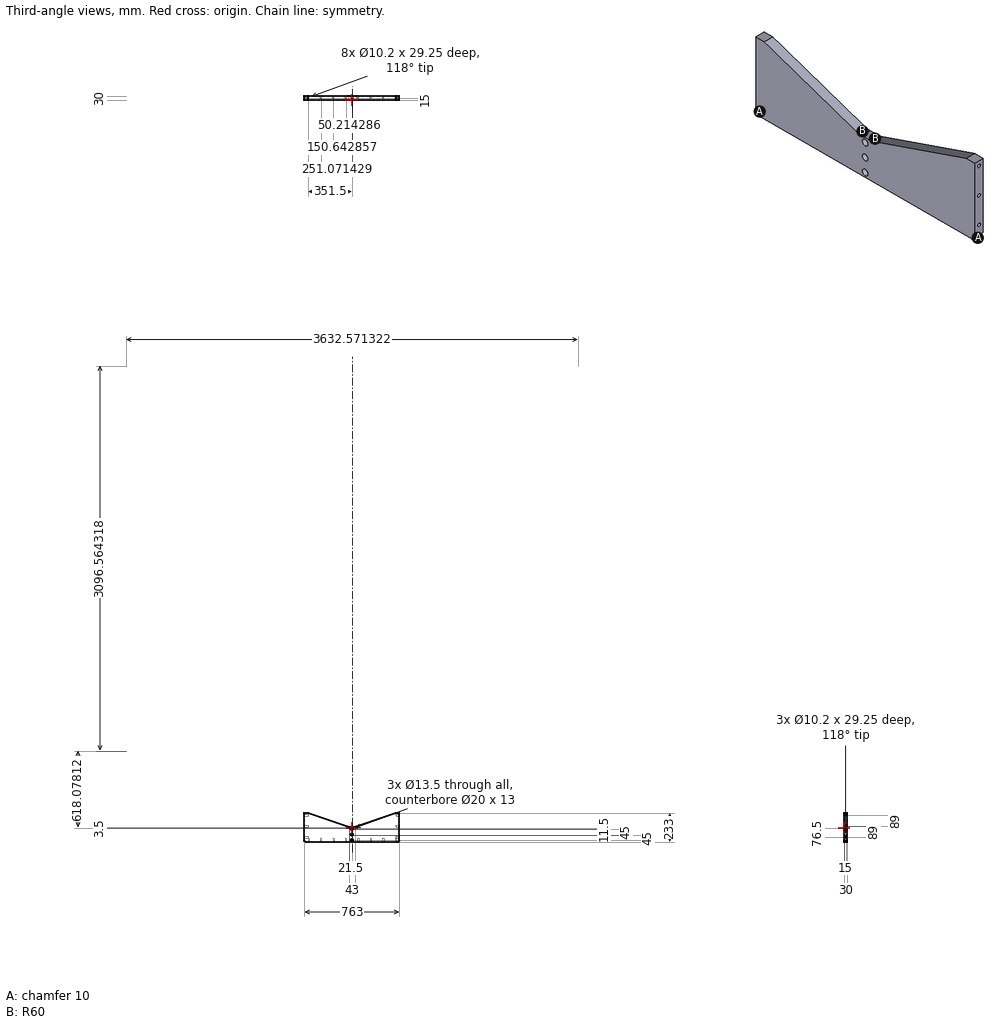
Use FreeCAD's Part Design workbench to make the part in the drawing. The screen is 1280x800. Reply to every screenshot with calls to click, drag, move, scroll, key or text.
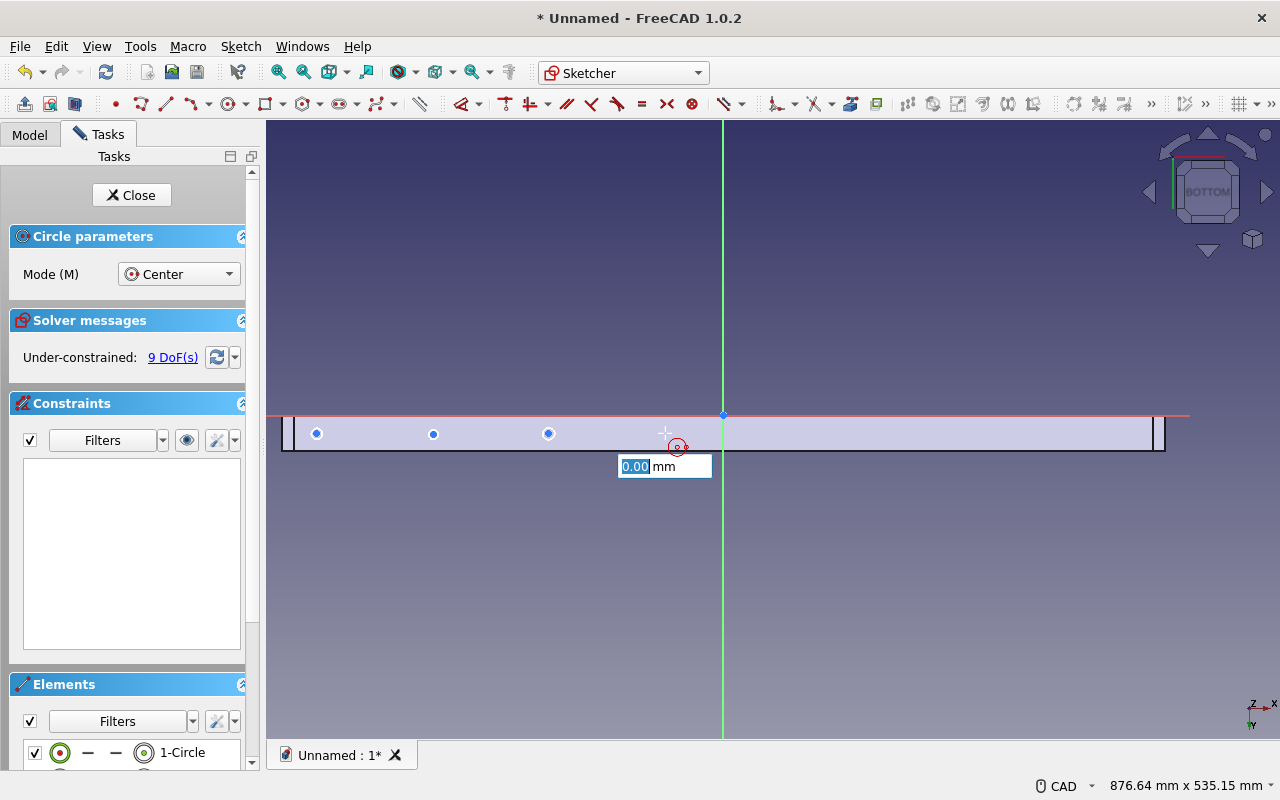
scroll(669, 437, up, 5)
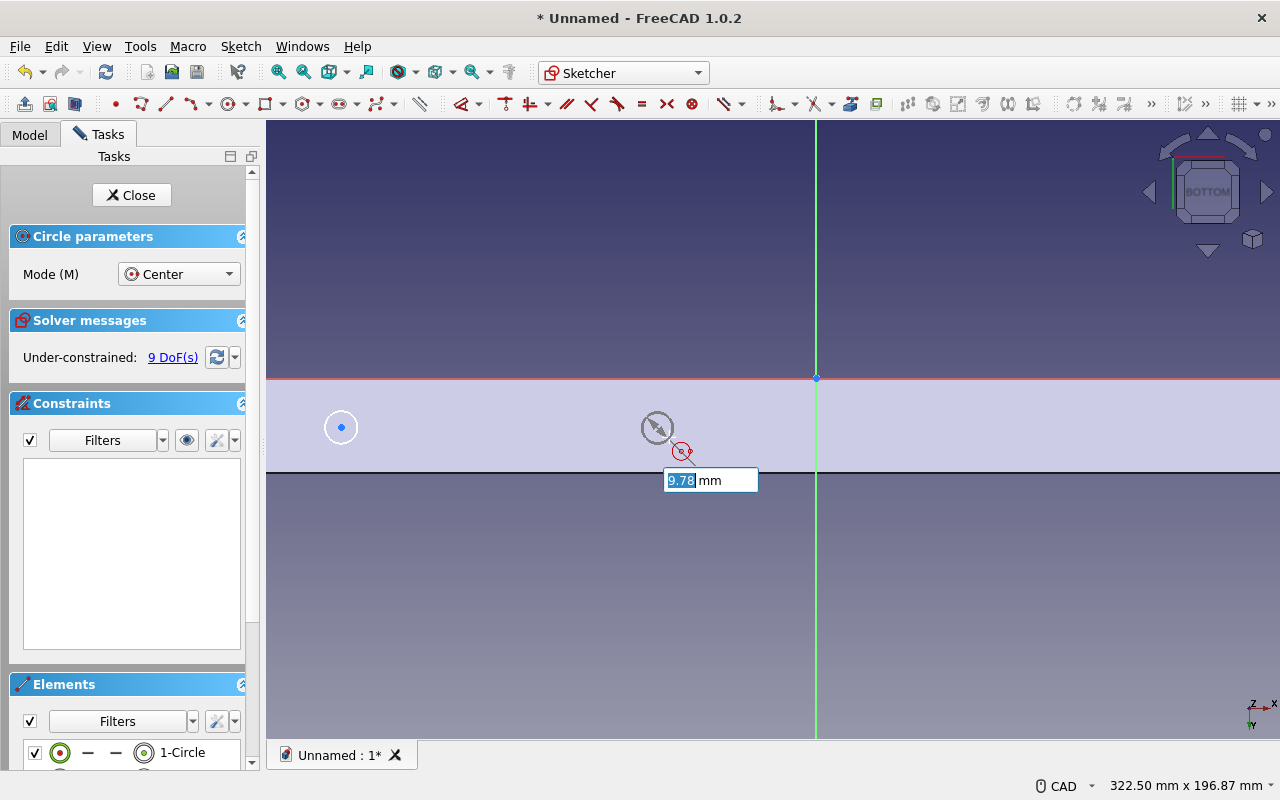
click(670, 437)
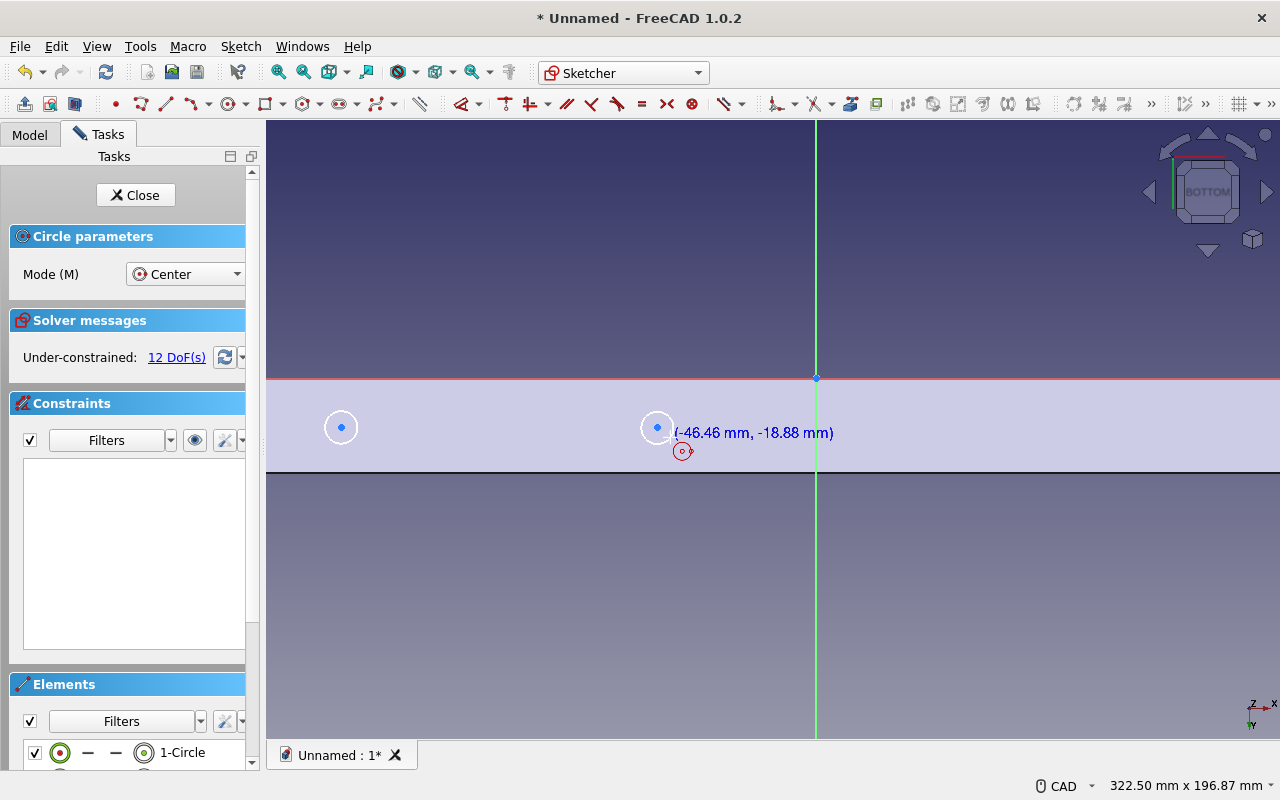
scroll(974, 426, up, 2)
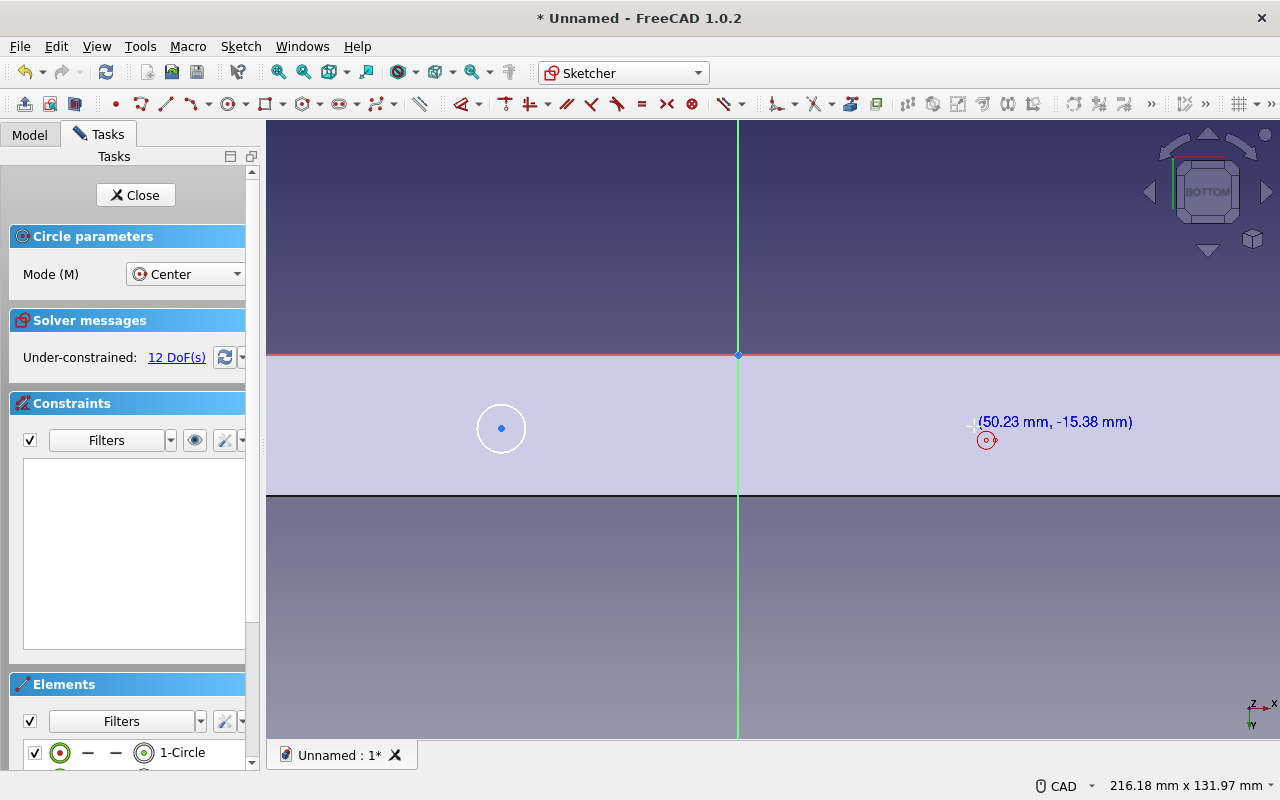
scroll(698, 435, down, 9)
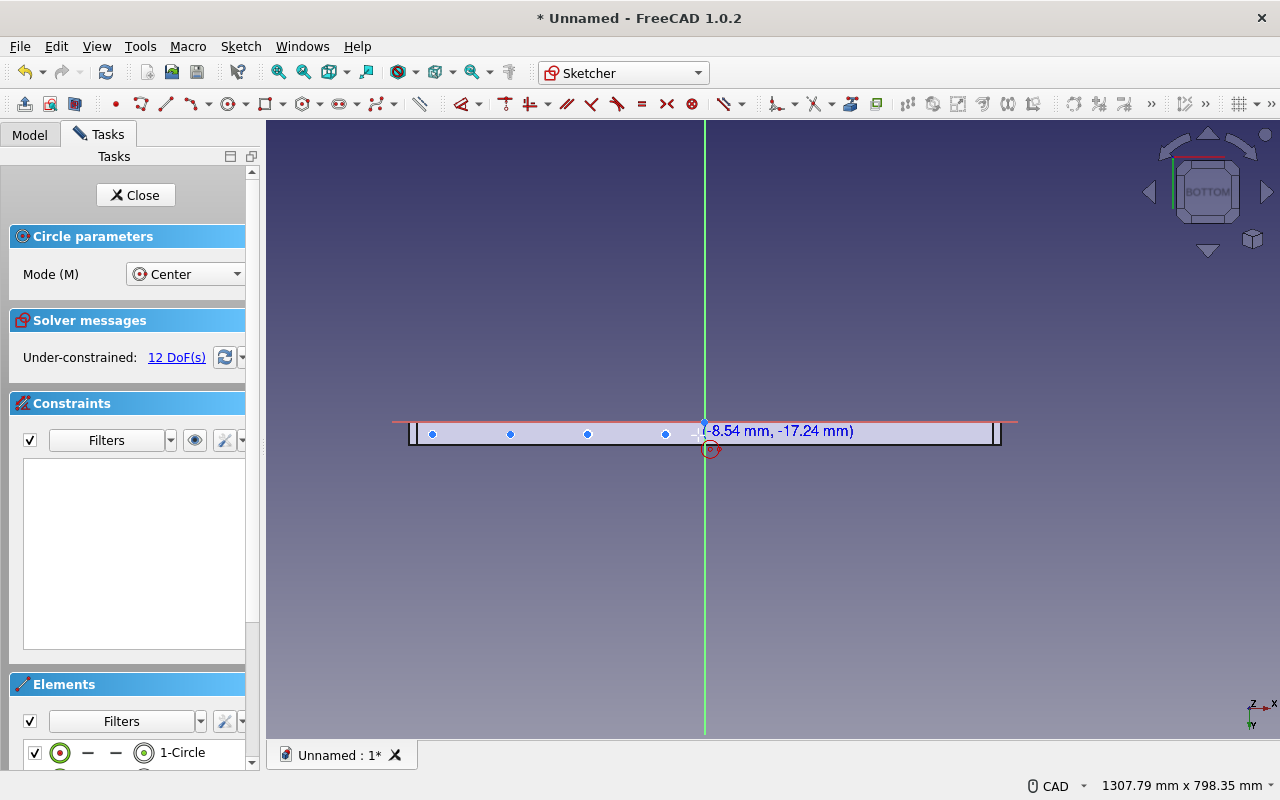
scroll(744, 434, up, 2)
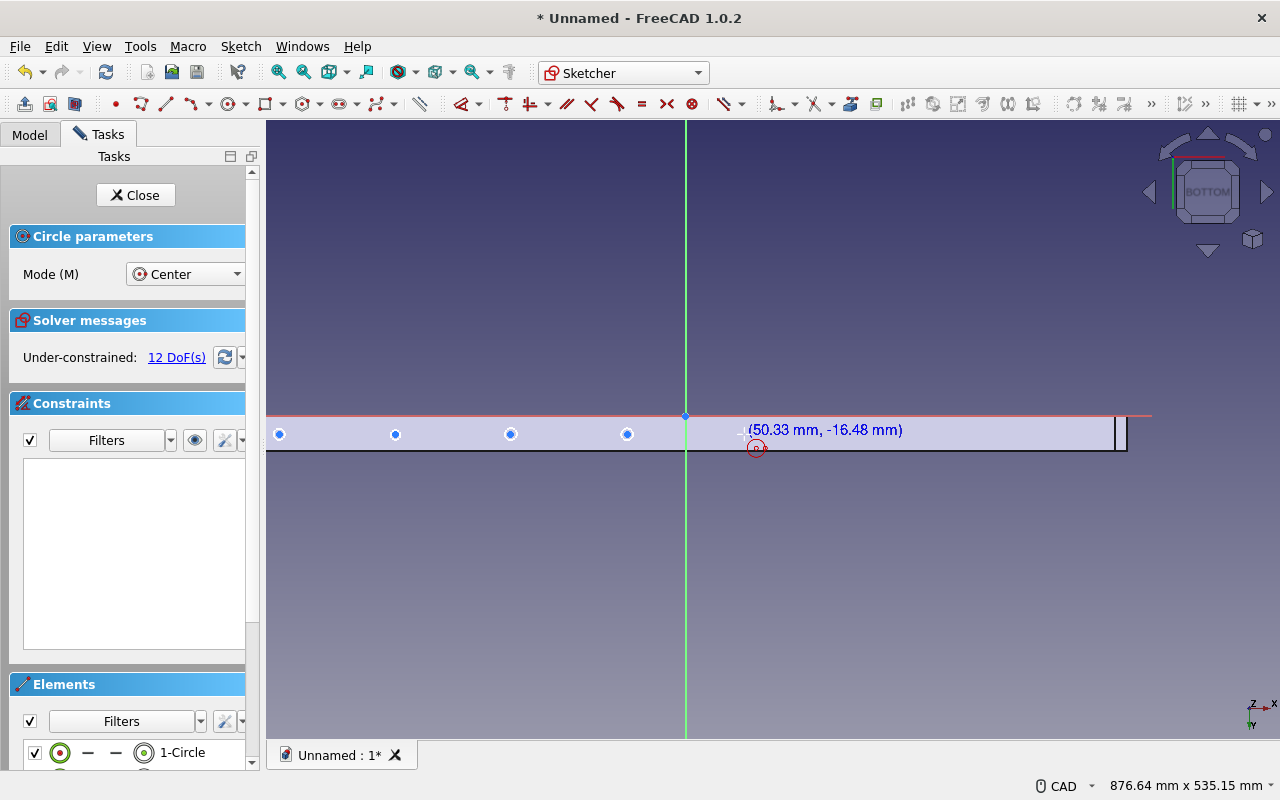
click(744, 434)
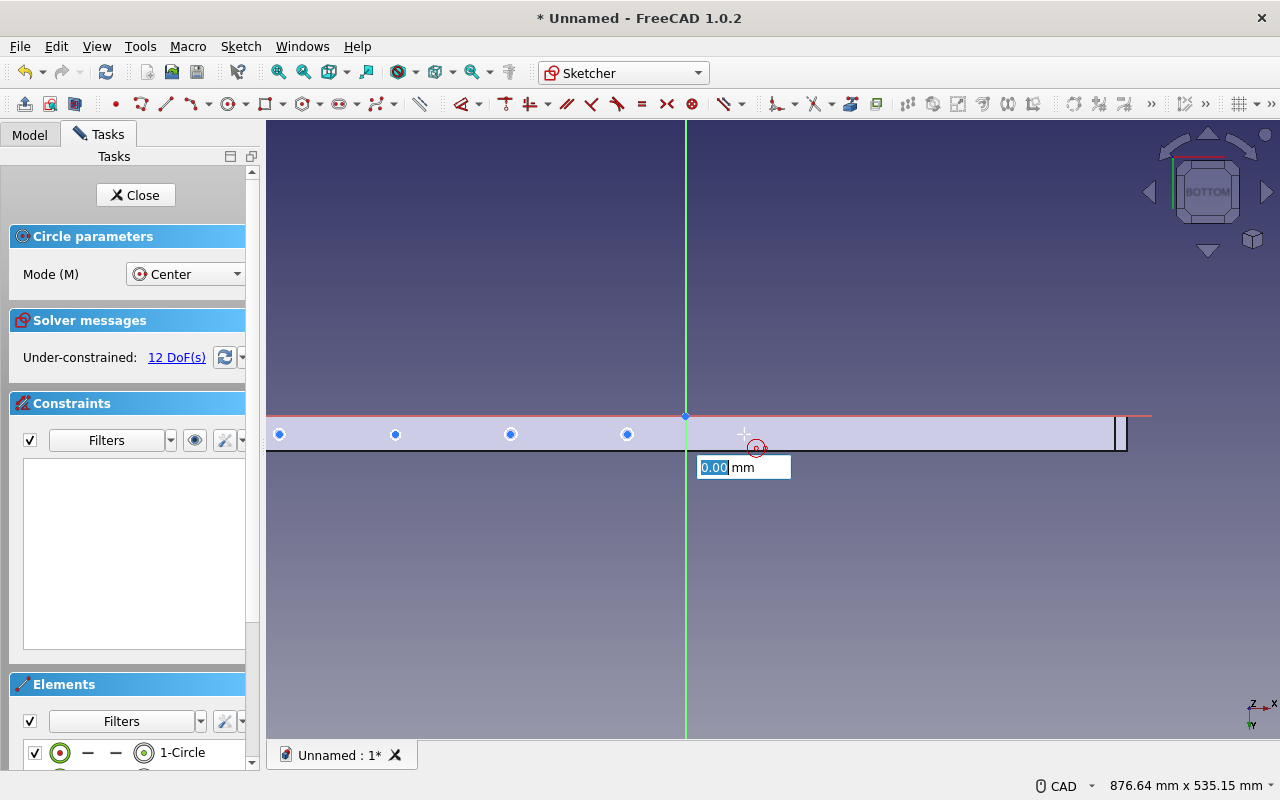
scroll(748, 438, up, 5)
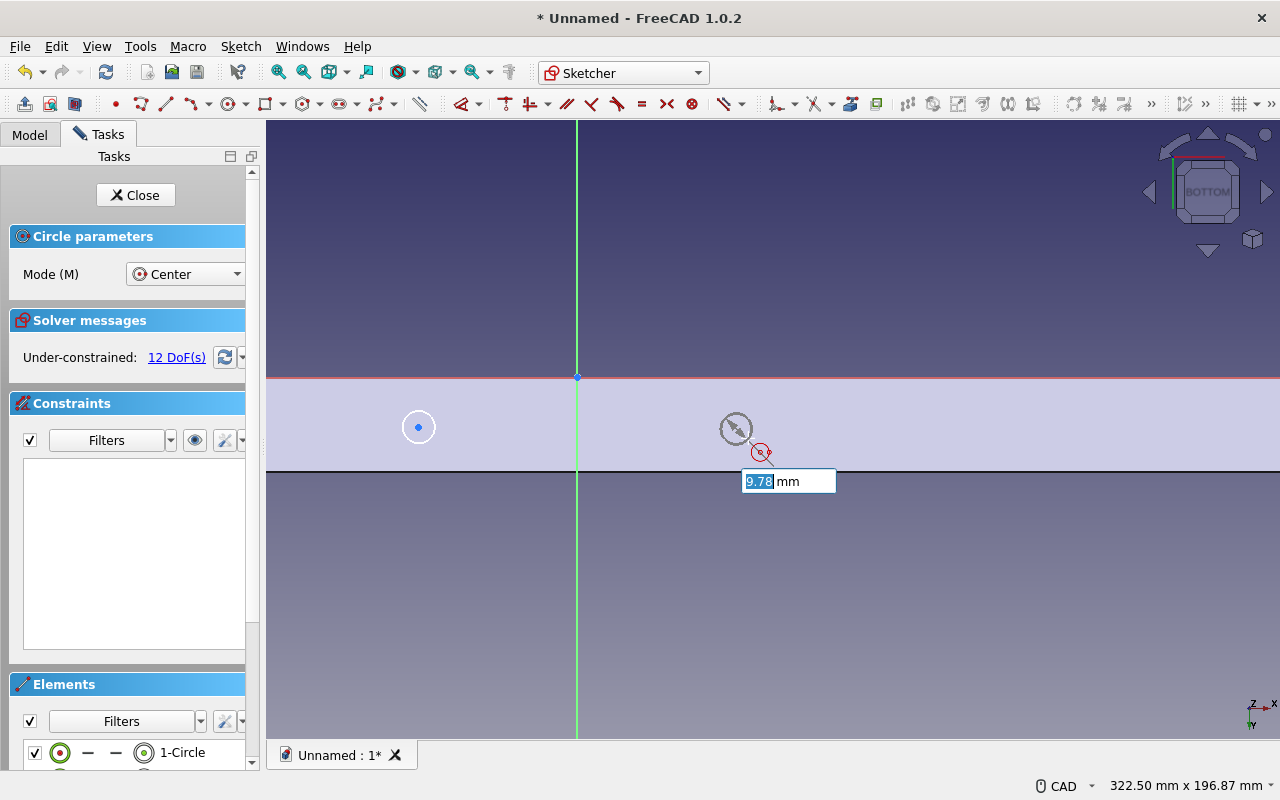
click(747, 436)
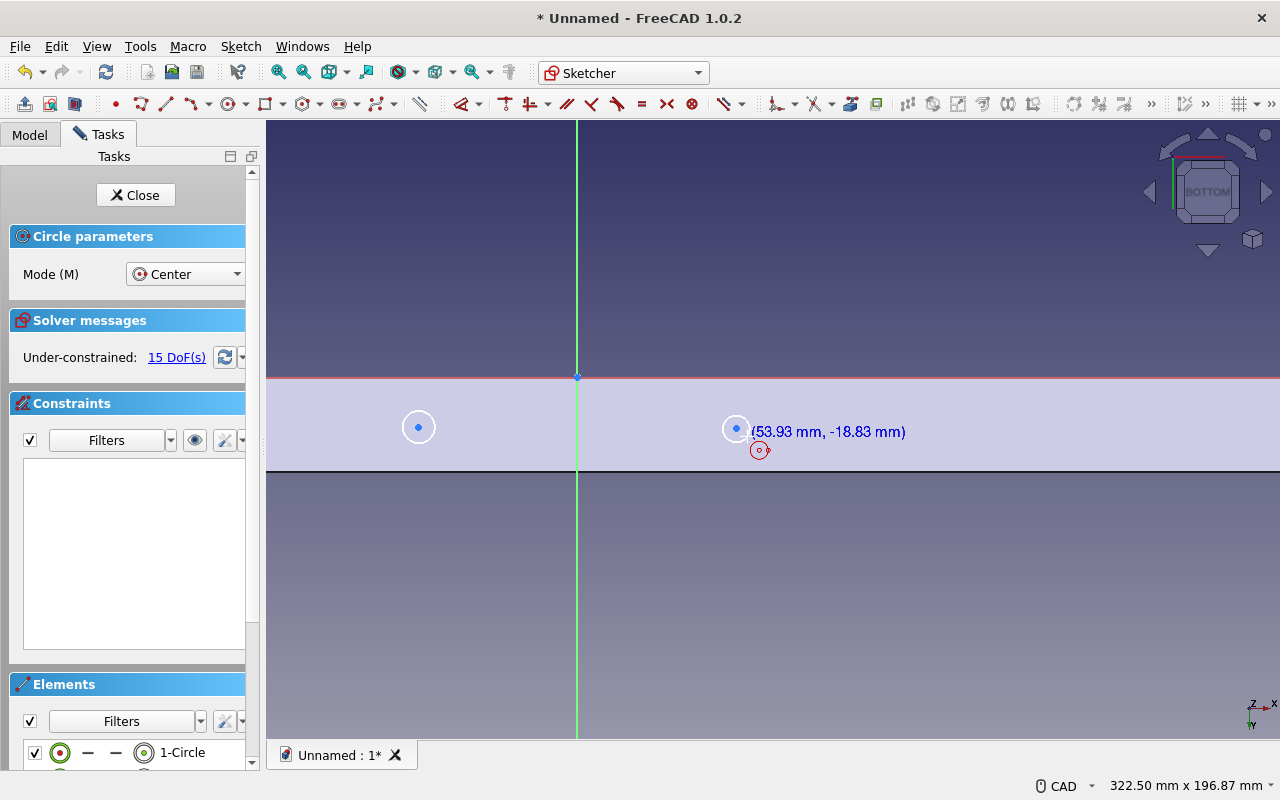
scroll(1051, 425, up, 2)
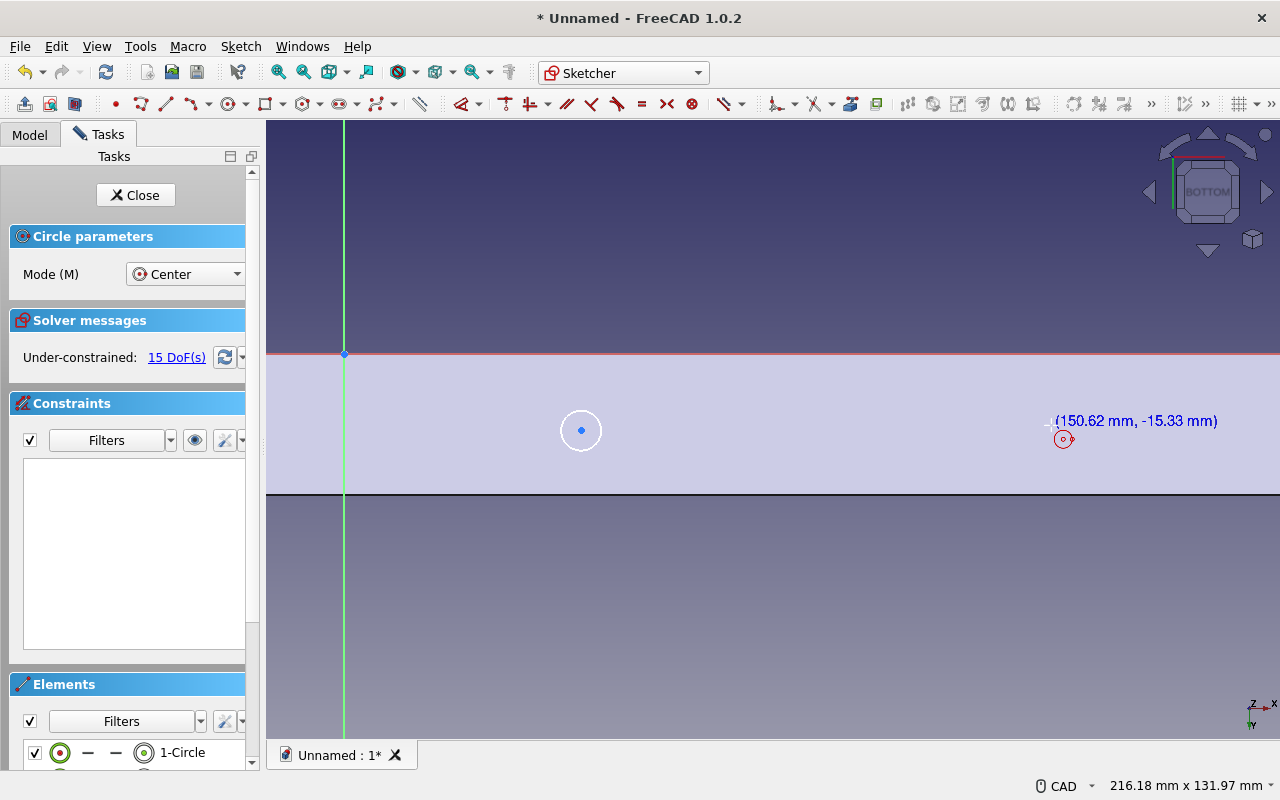
scroll(776, 435, down, 9)